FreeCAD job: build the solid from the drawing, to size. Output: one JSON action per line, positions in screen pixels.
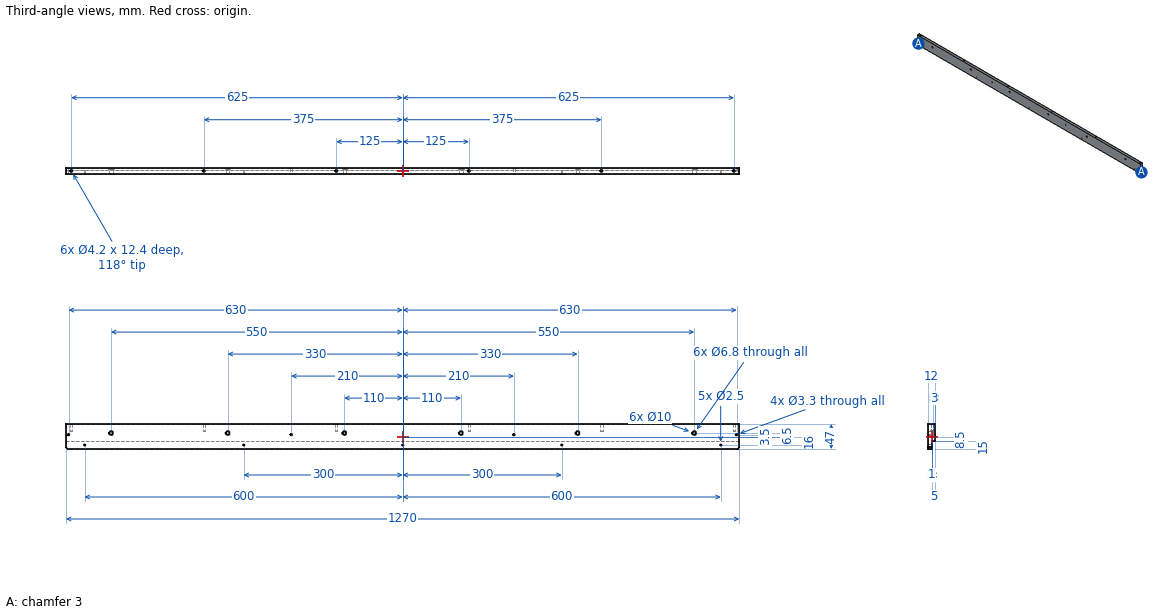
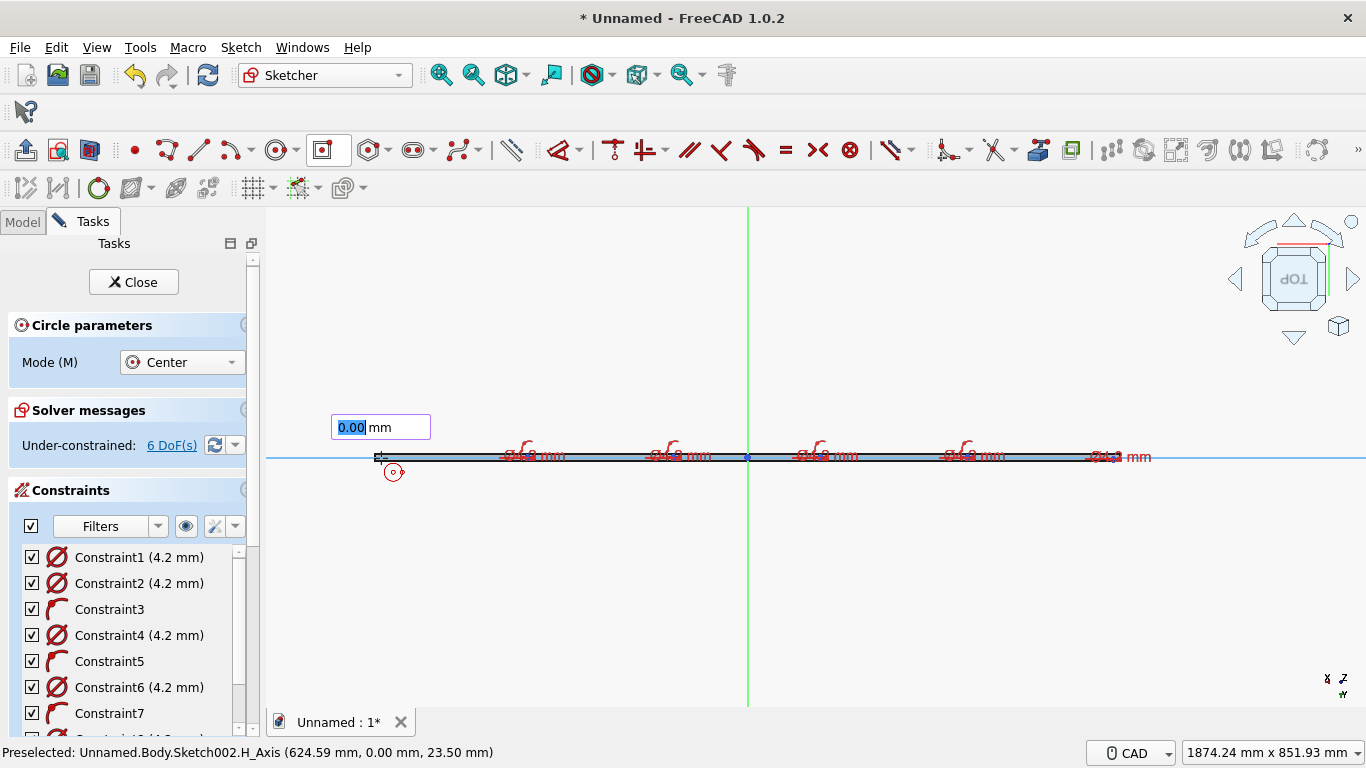
{"action": "scroll", "coordinate": [380, 459], "scroll_direction": "up", "scroll_amount": 14}
{"action": "mouse_move", "coordinate": [384, 451]}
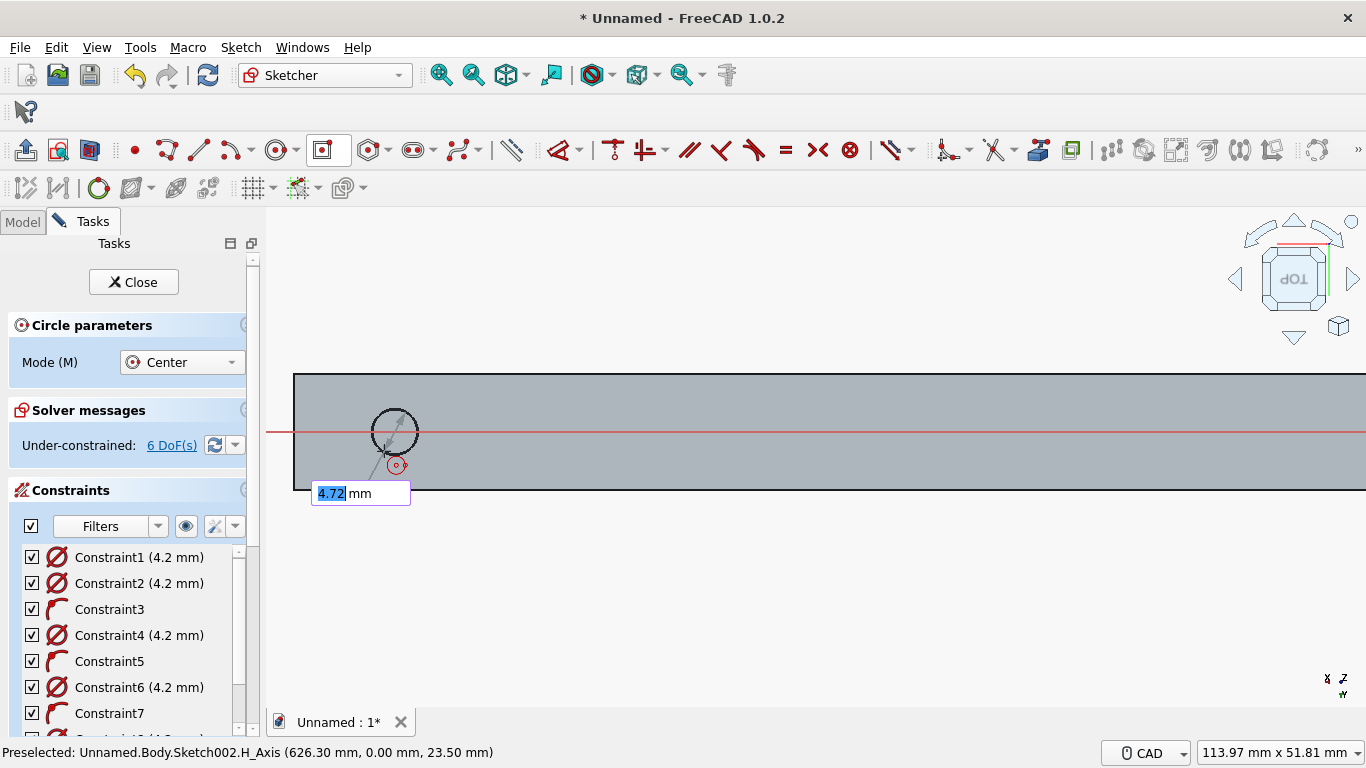
{"action": "type", "text": "4.2"}
{"action": "key", "text": "Return"}
{"action": "key", "text": "Escape"}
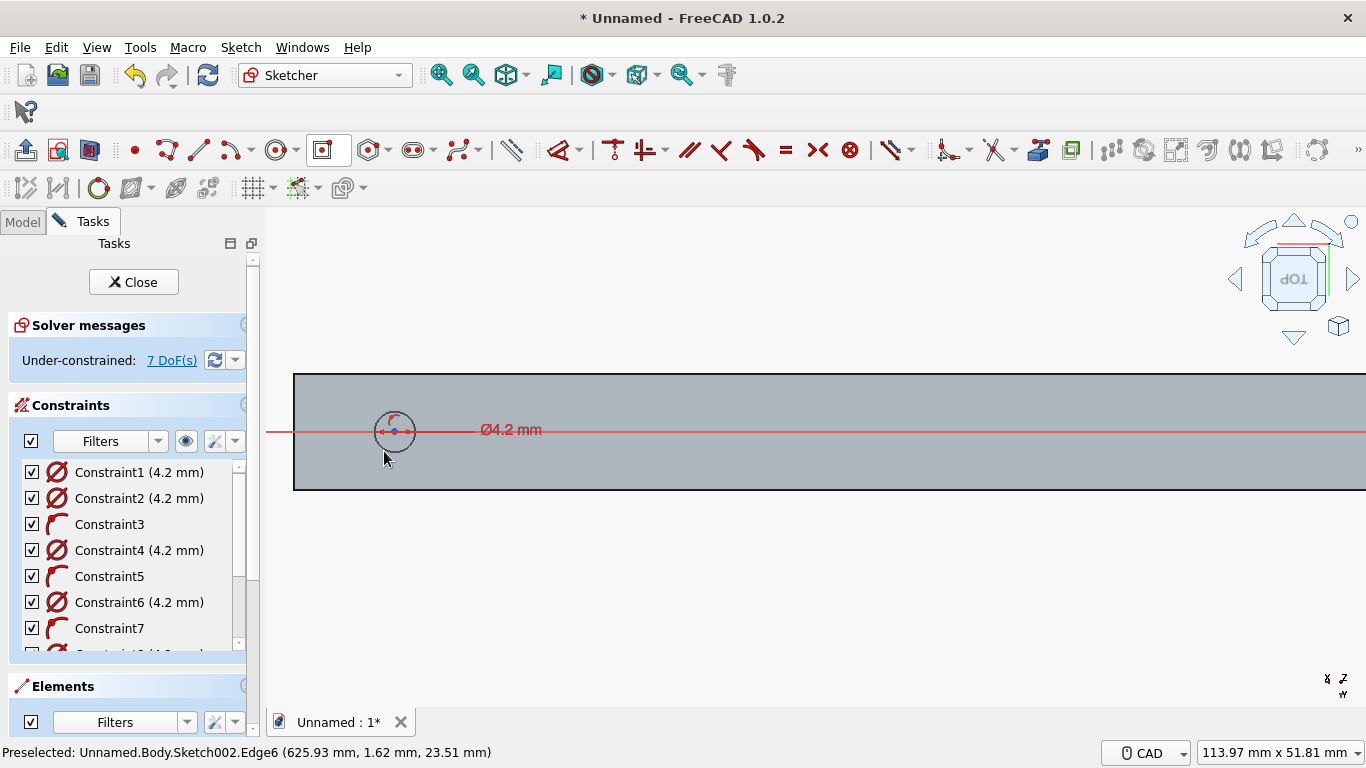
{"action": "scroll", "coordinate": [450, 458], "scroll_direction": "down", "scroll_amount": 15}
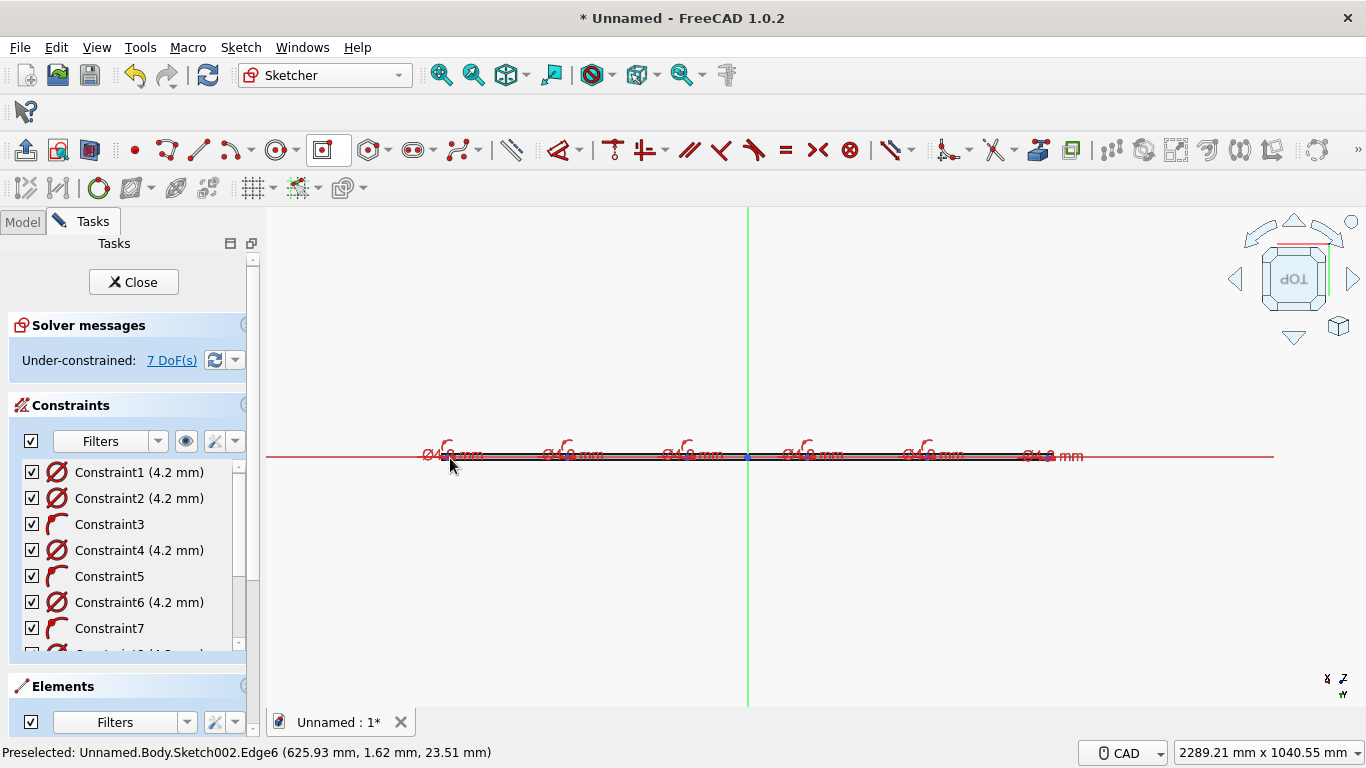
{"action": "left_click", "coordinate": [1048, 458]}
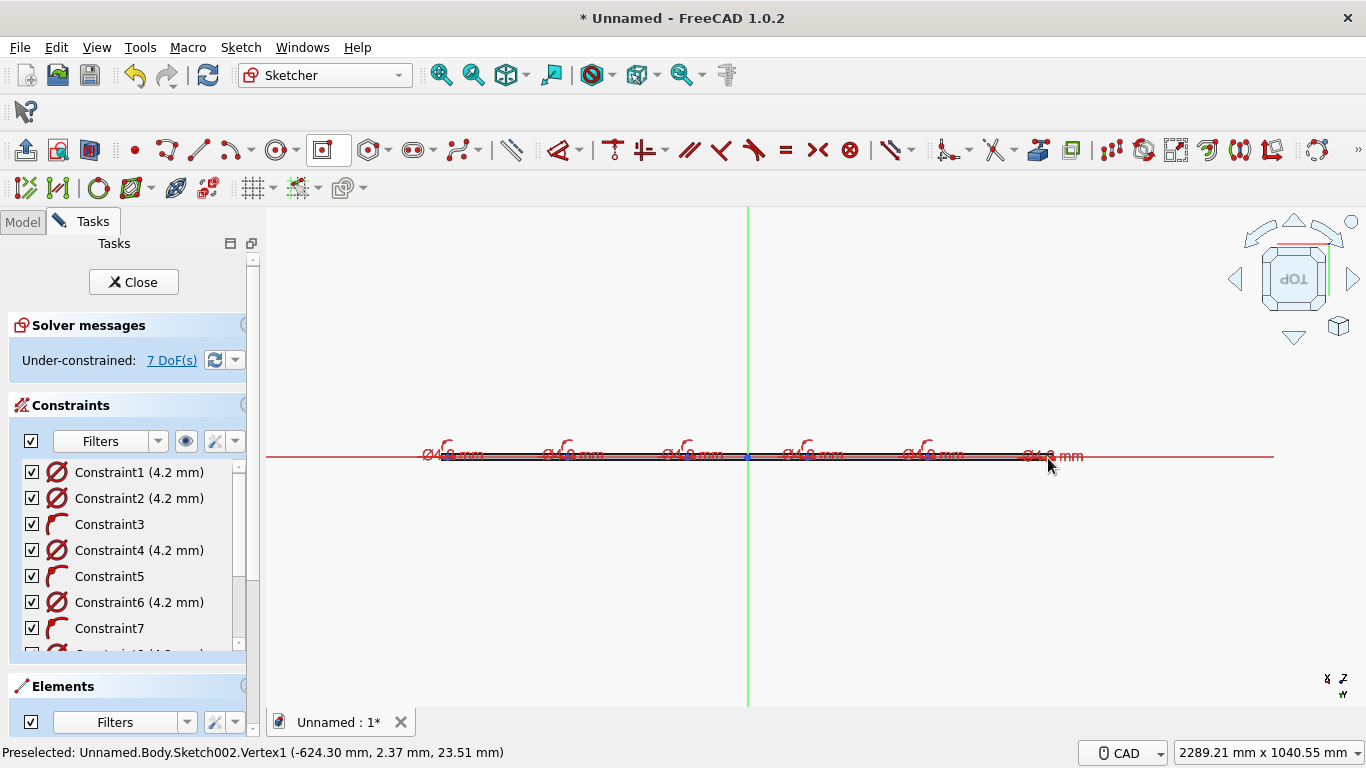
{"action": "left_click", "coordinate": [359, 457]}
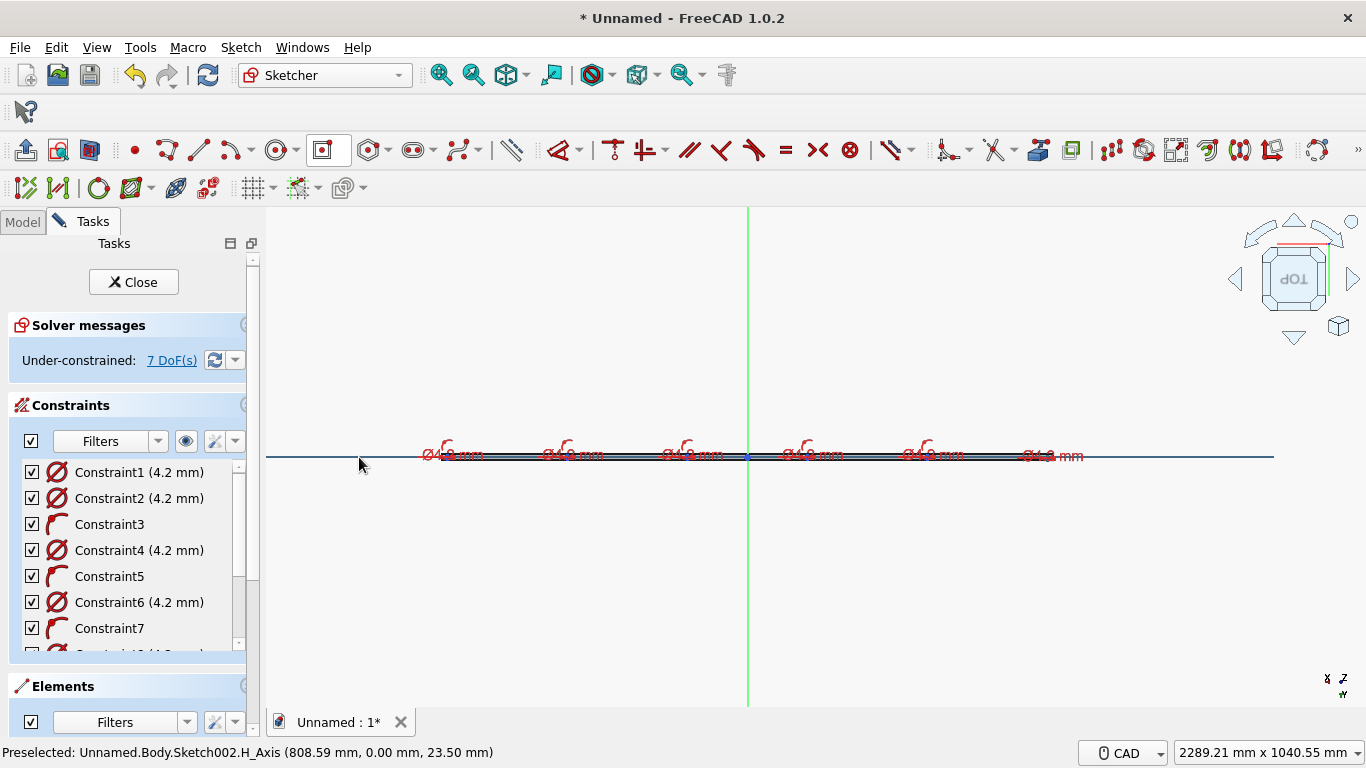
{"action": "left_click", "coordinate": [614, 150]}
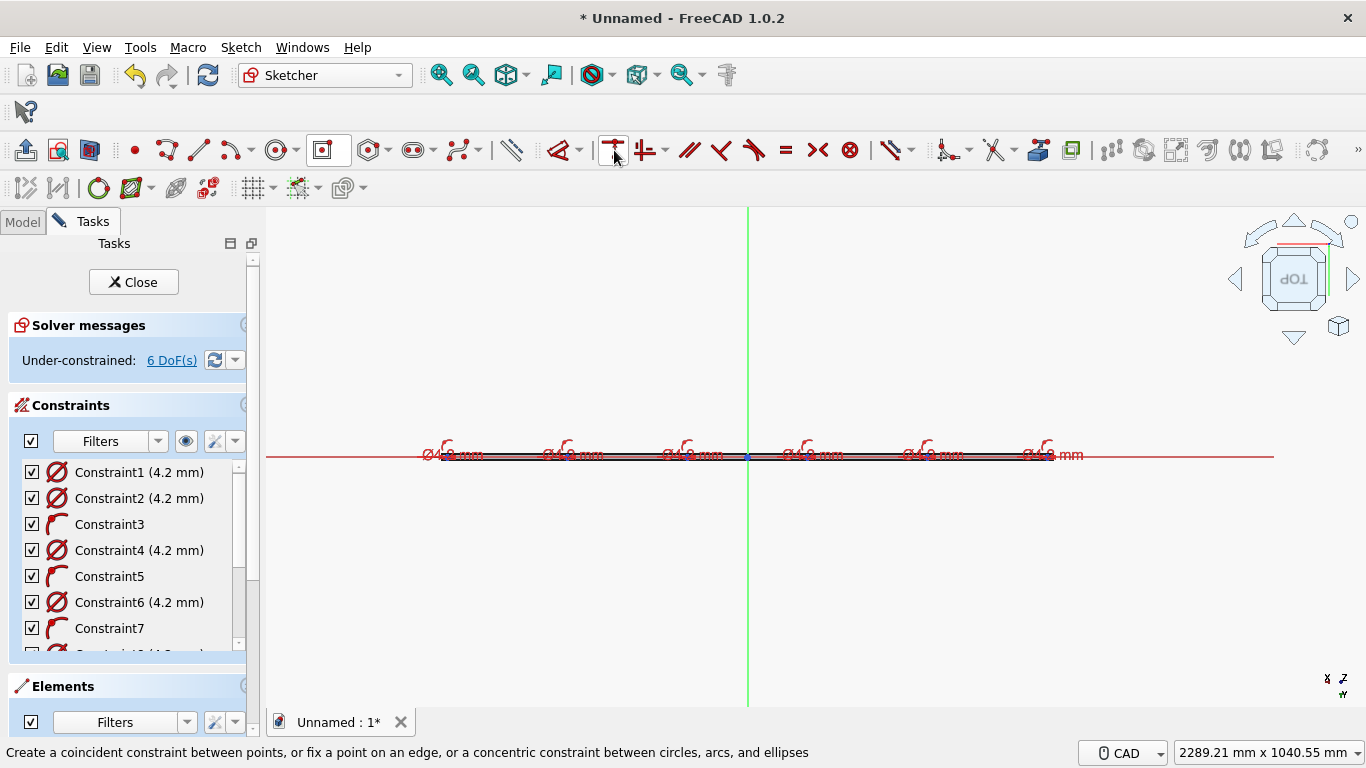
{"action": "left_click", "coordinate": [558, 150]}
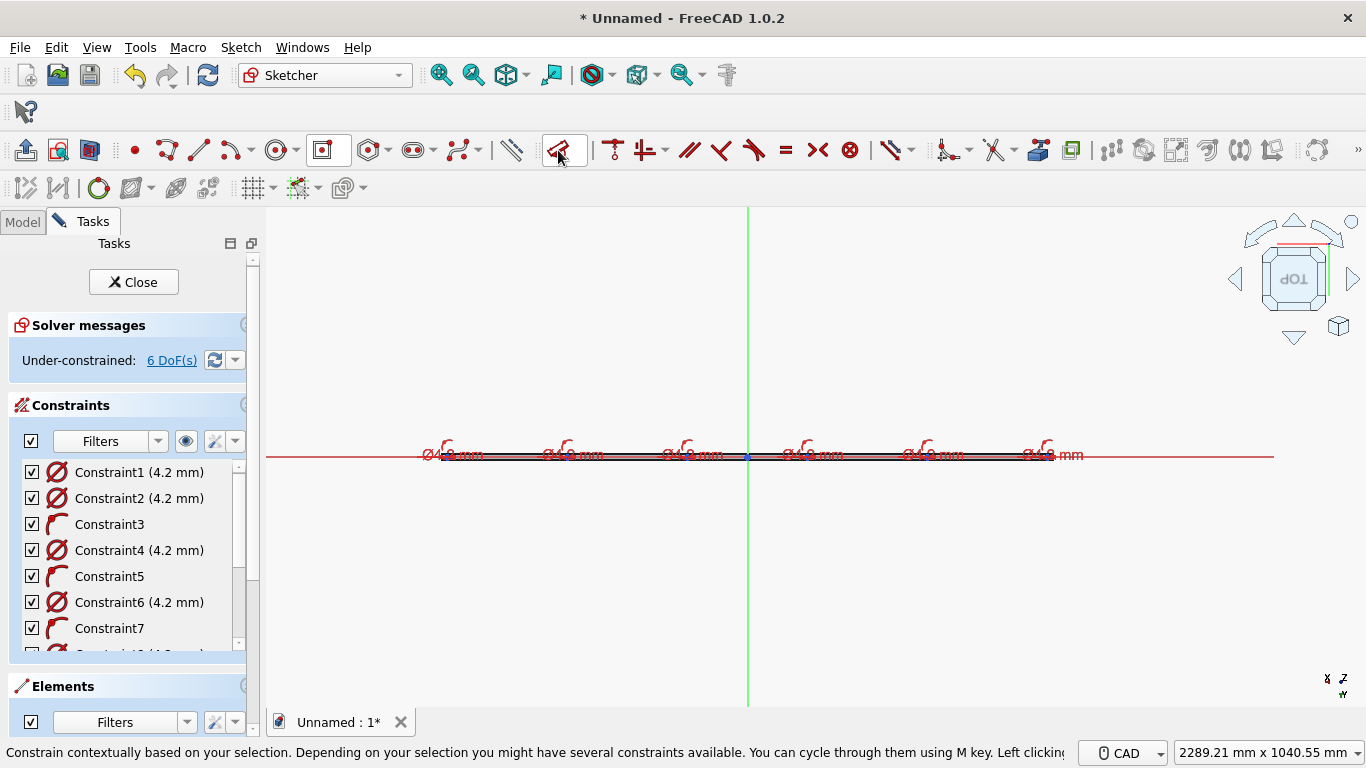
{"action": "left_click", "coordinate": [1048, 457]}
{"action": "left_click", "coordinate": [898, 491]}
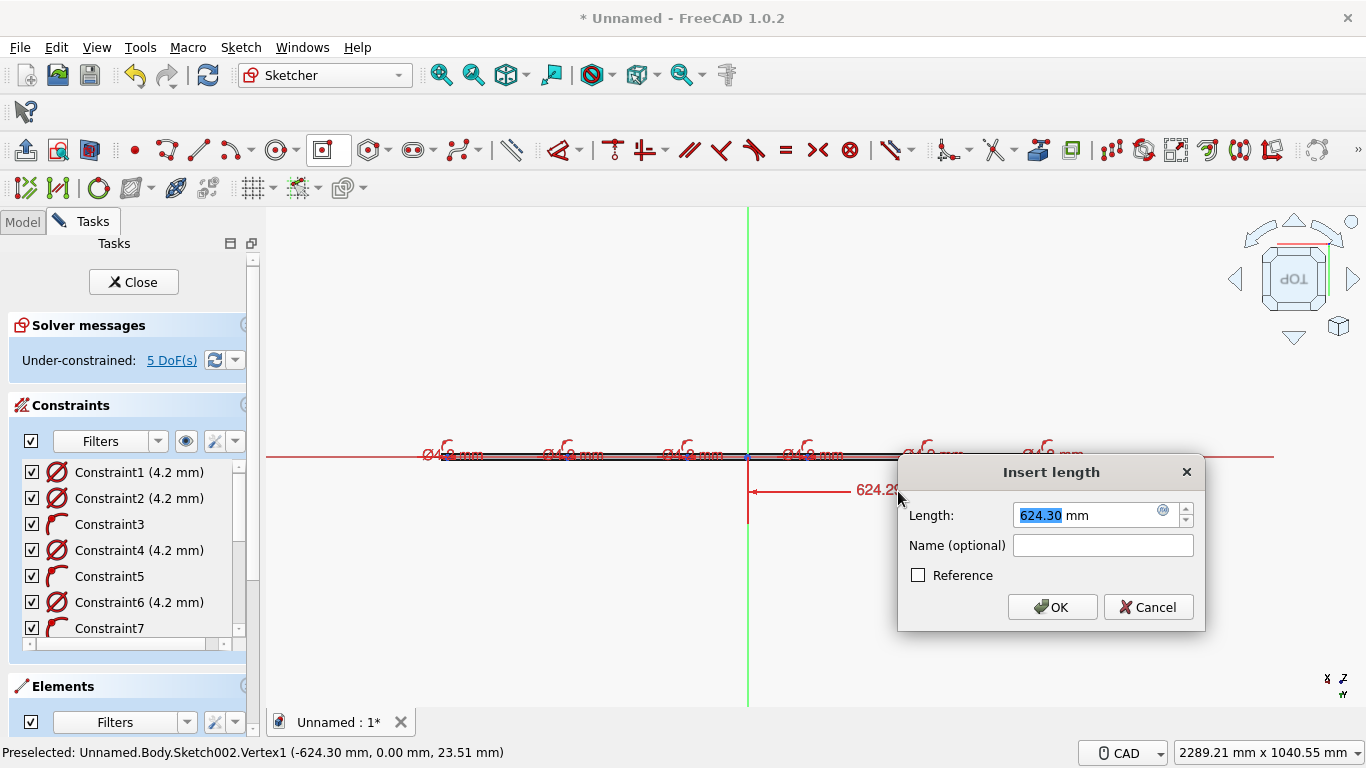
{"action": "type", "text": "625"}
{"action": "key", "text": "Return"}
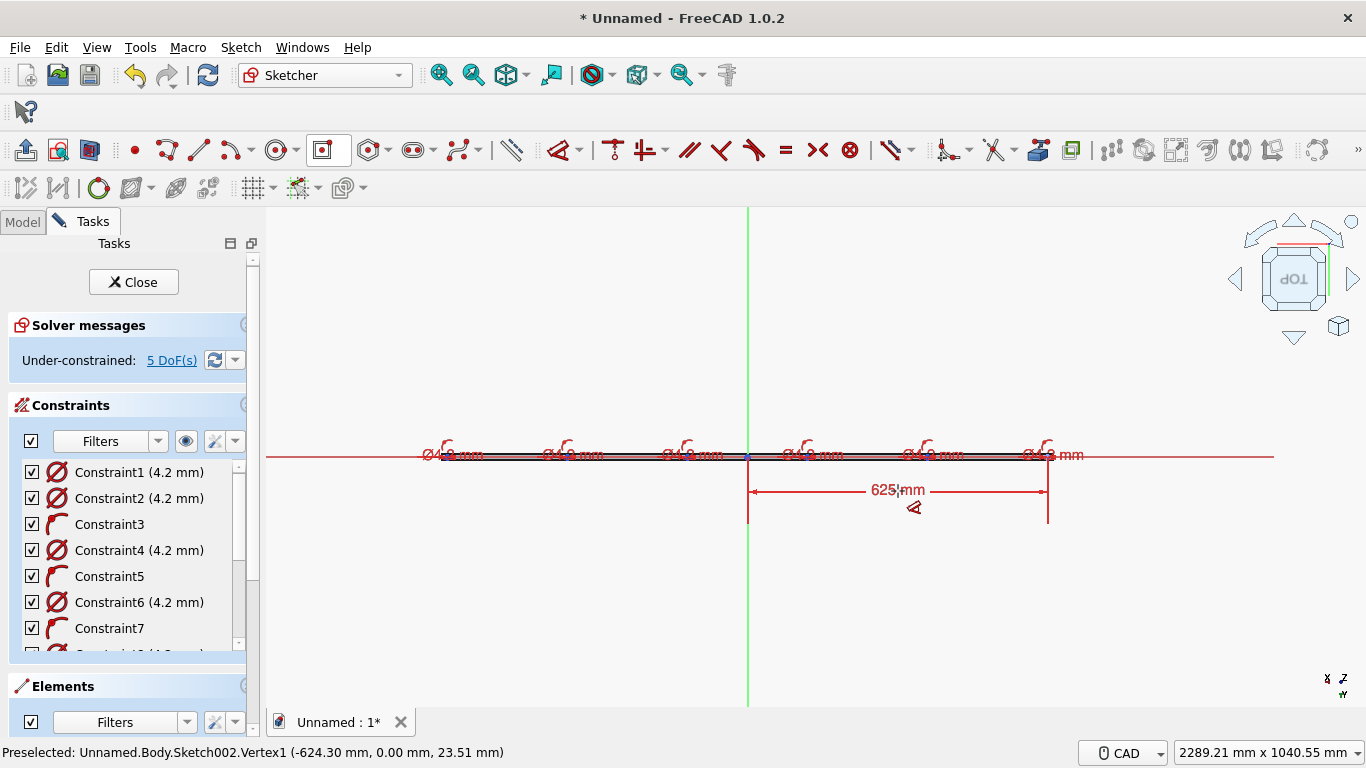
{"action": "left_click", "coordinate": [928, 457]}
{"action": "left_click", "coordinate": [796, 491]}